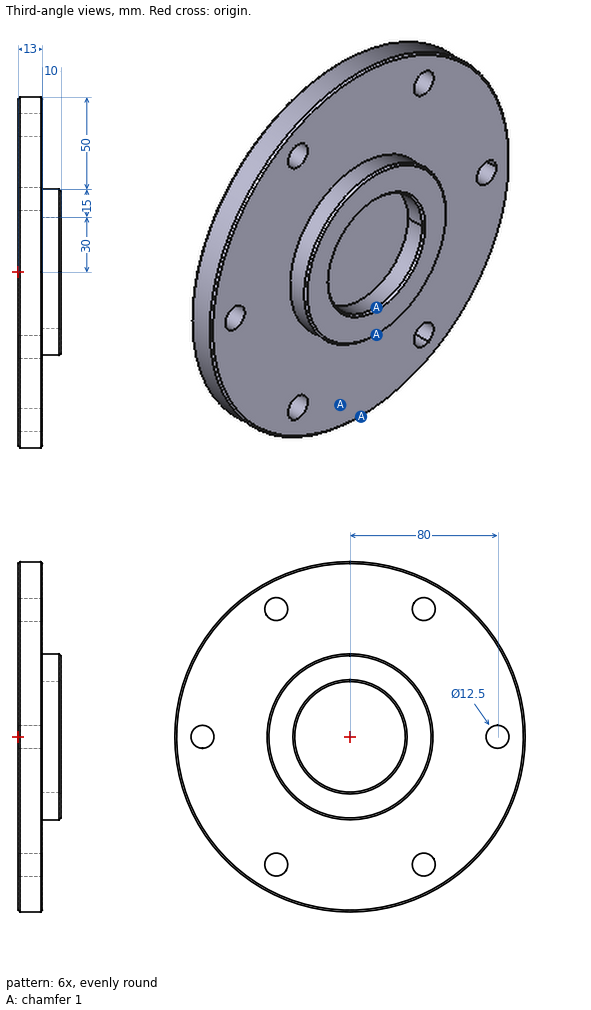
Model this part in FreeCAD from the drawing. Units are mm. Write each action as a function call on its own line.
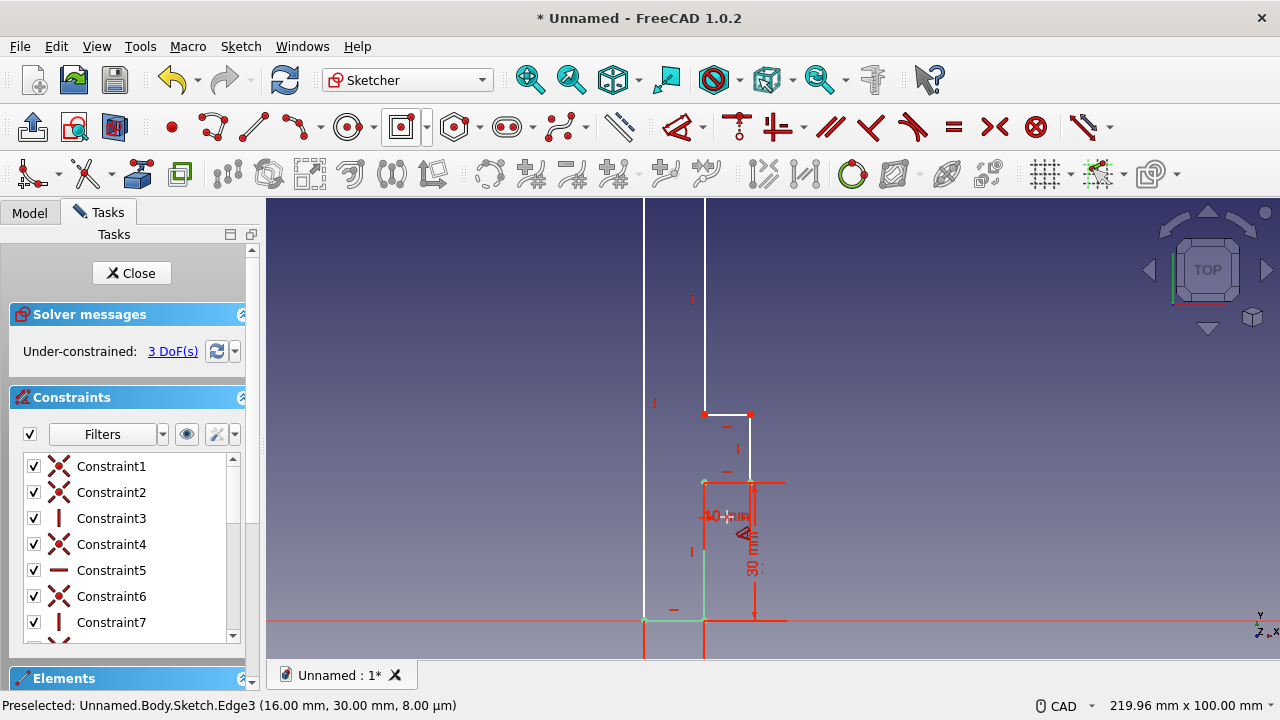
click(750, 462)
click(784, 449)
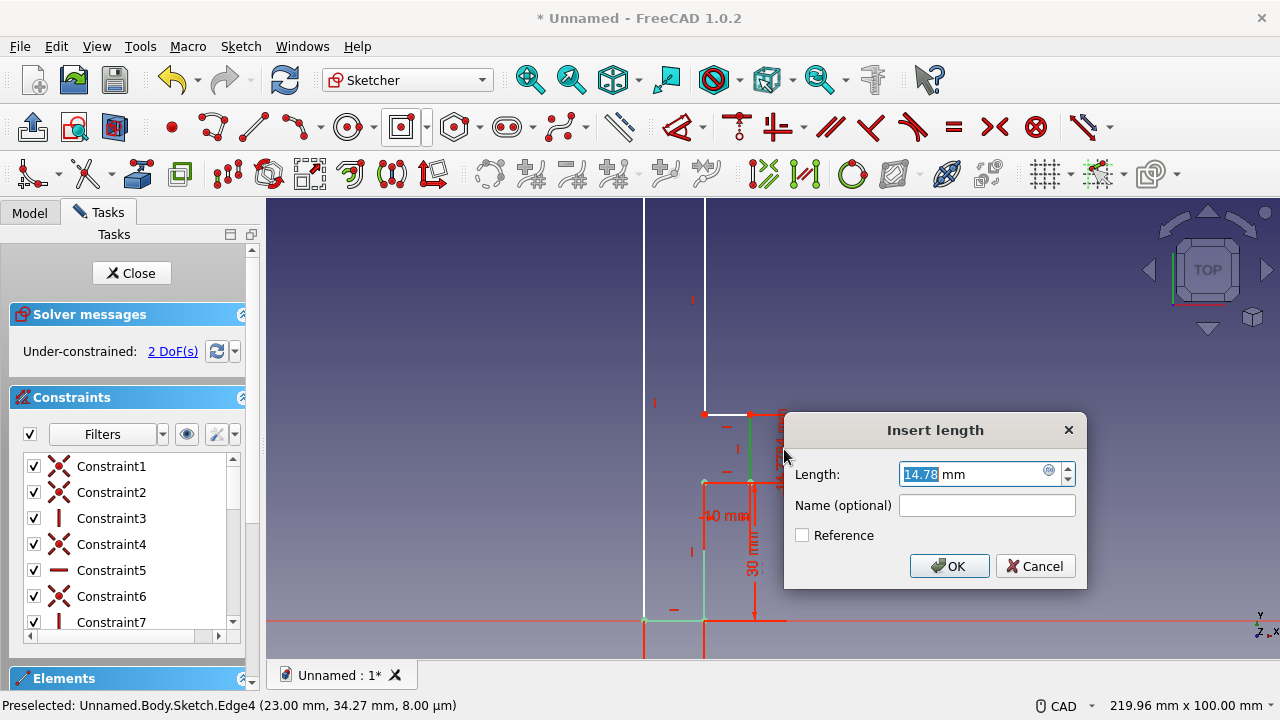
text(15)
key(Return)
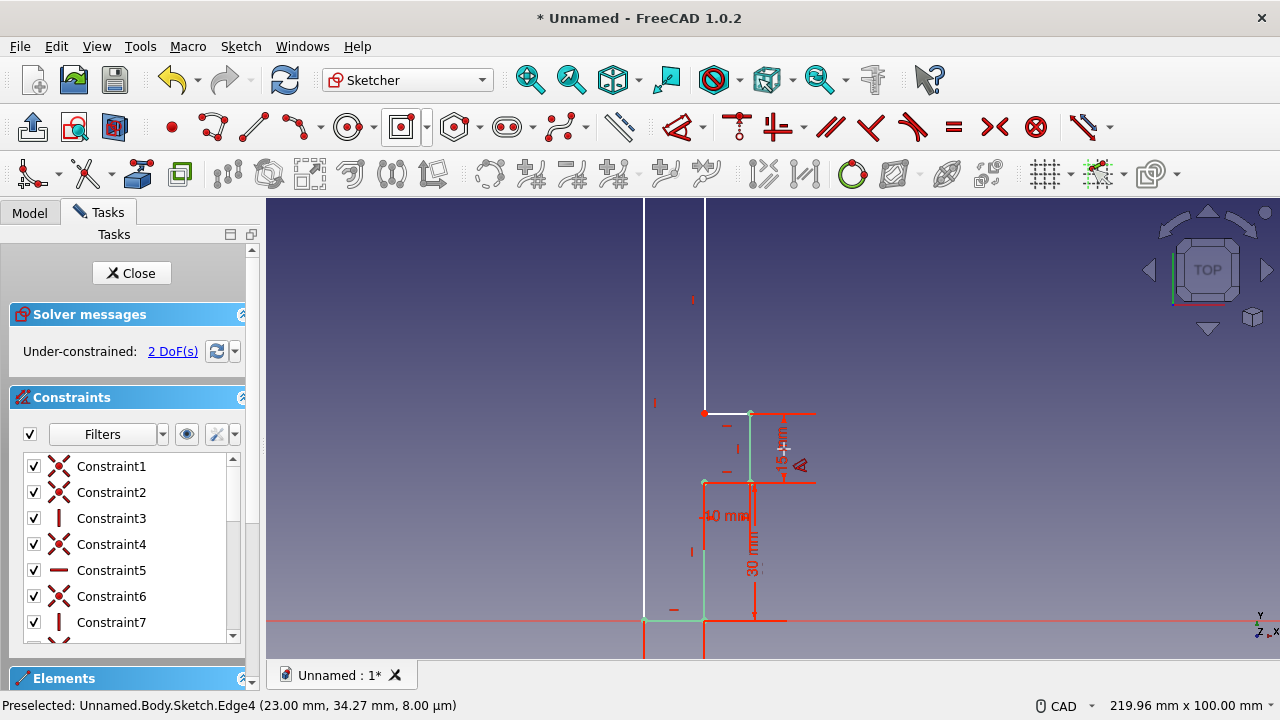
click(737, 414)
click(712, 448)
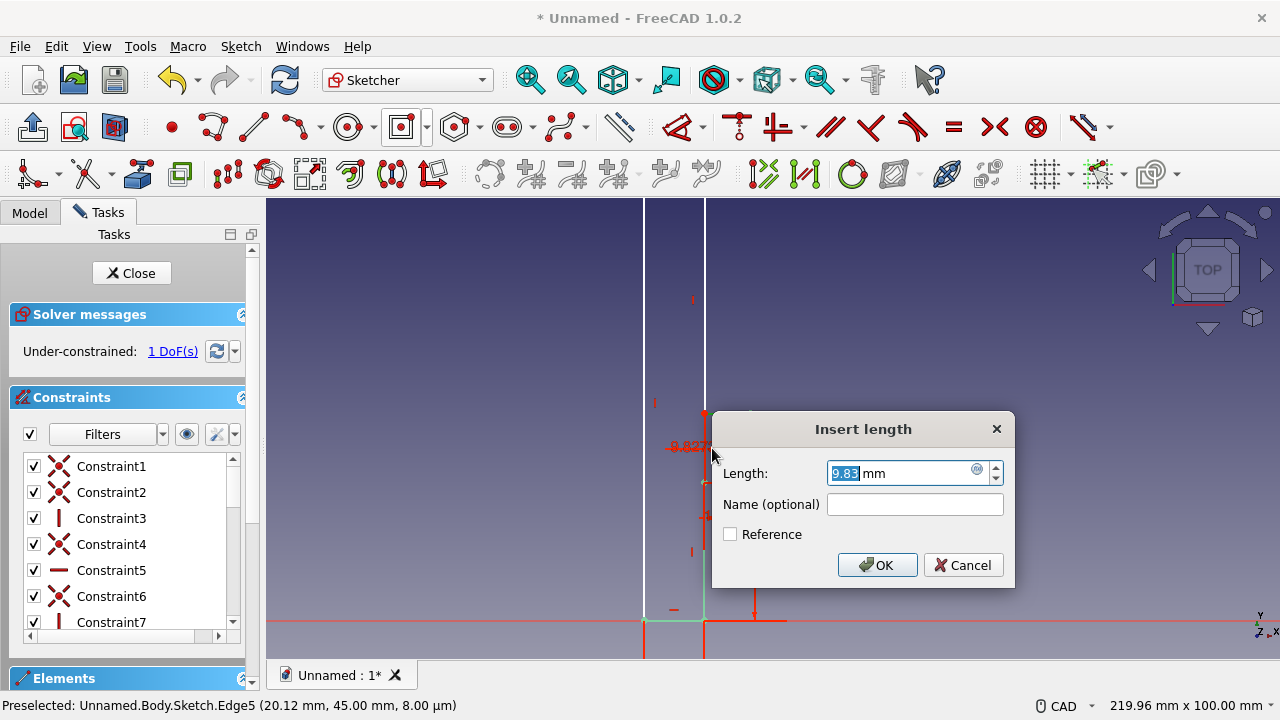
text(10)
key(Return)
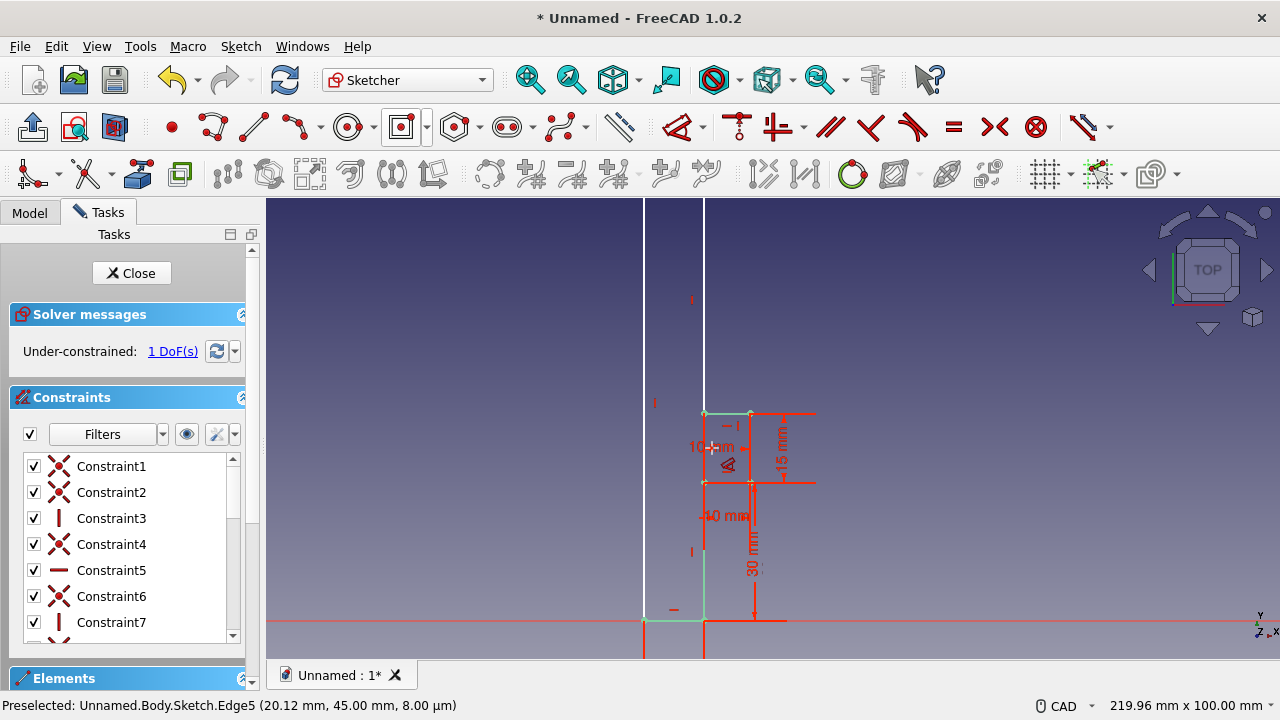
click(704, 345)
click(738, 320)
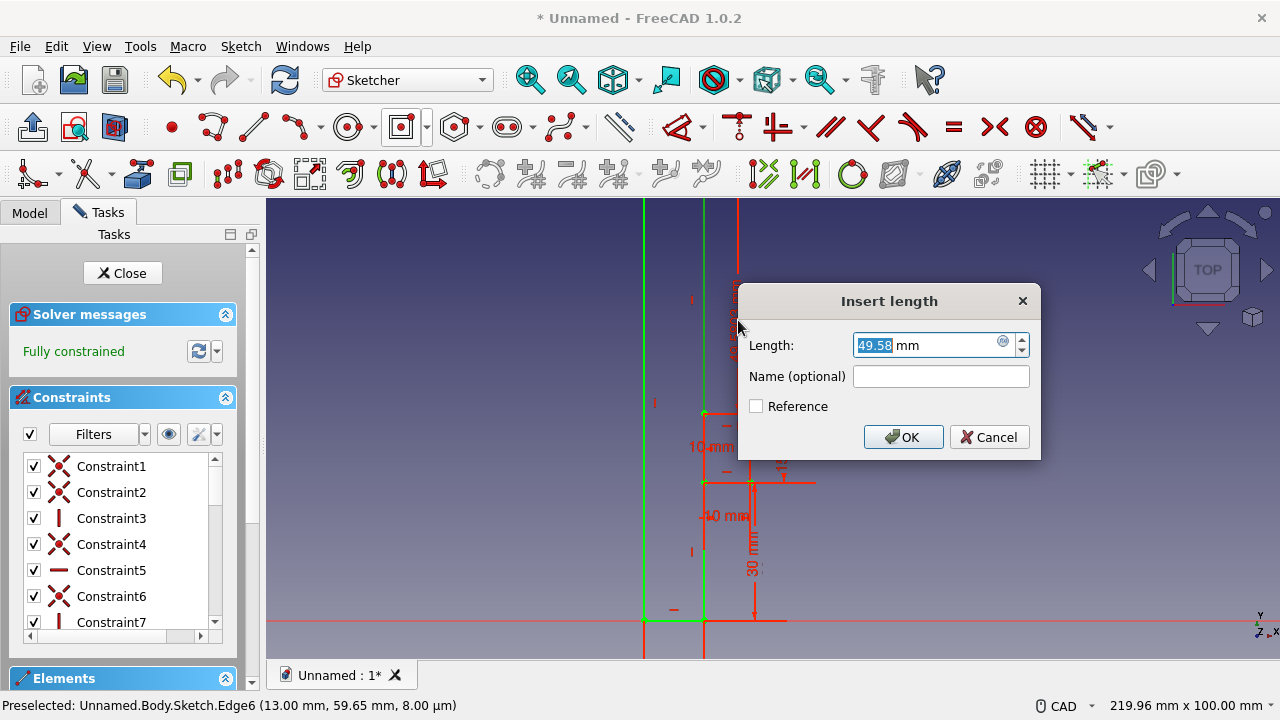
text(50)
key(Return)
key(Escape)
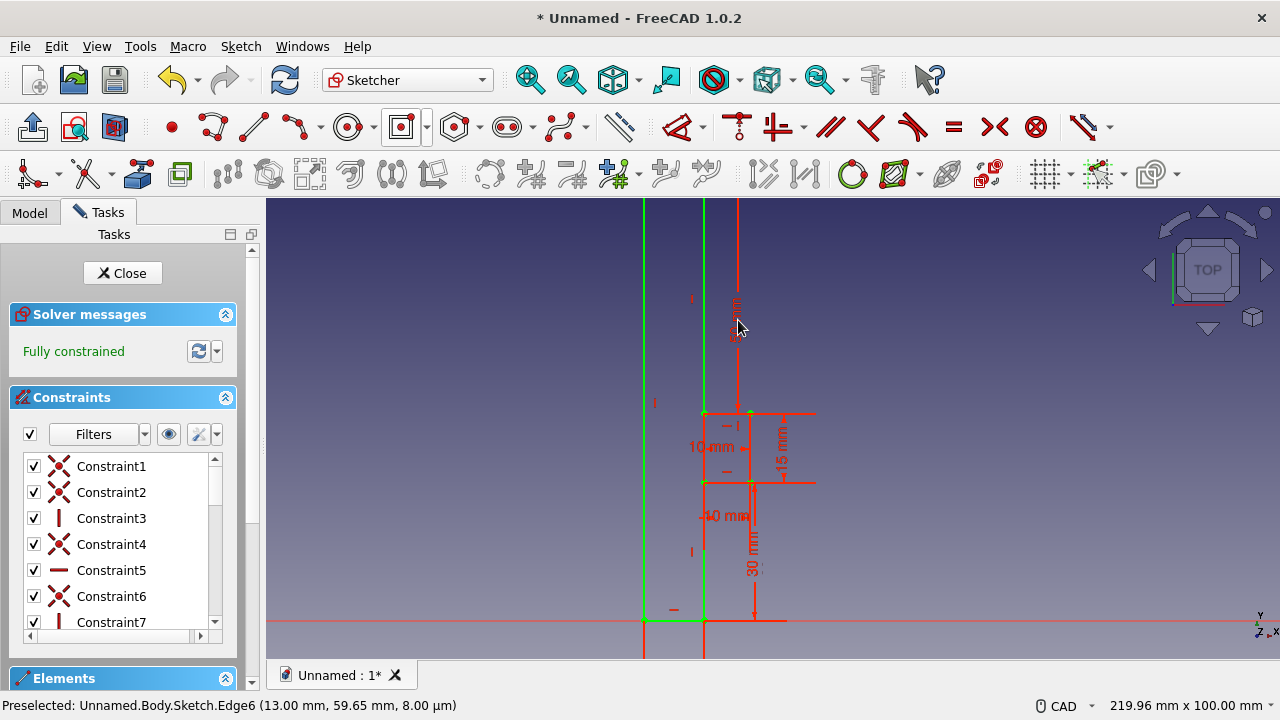
click(123, 273)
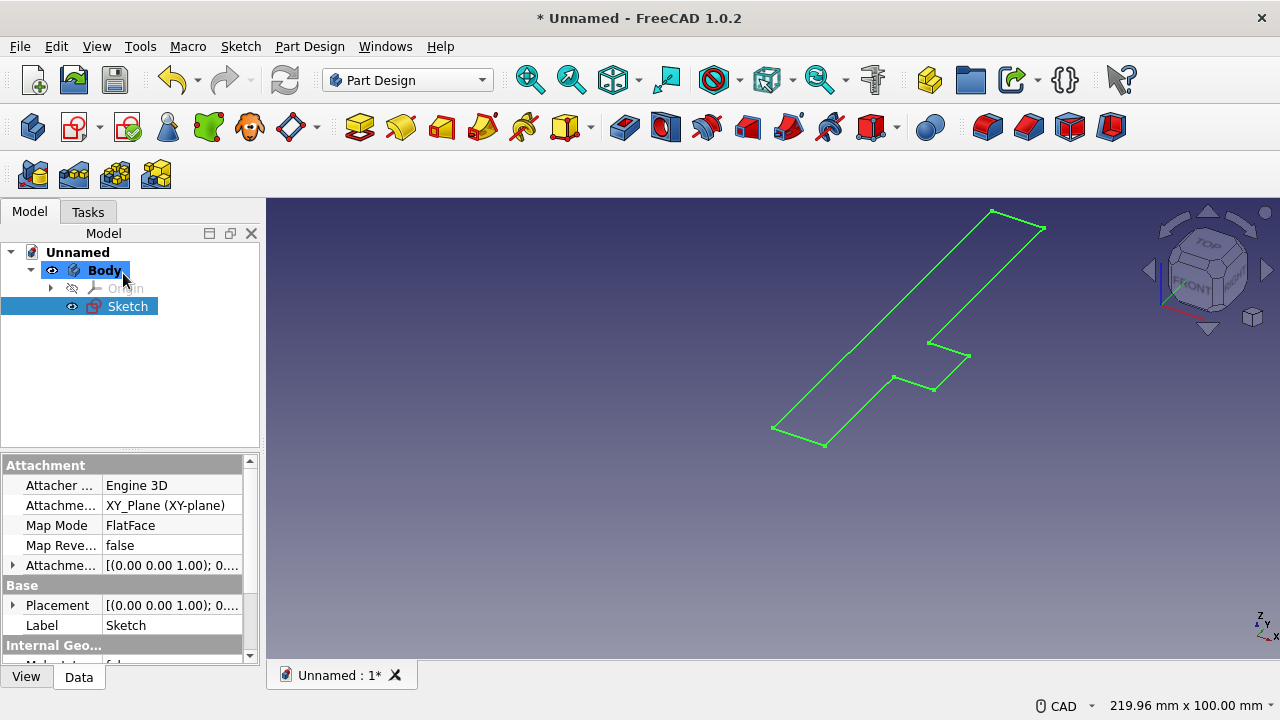
click(401, 128)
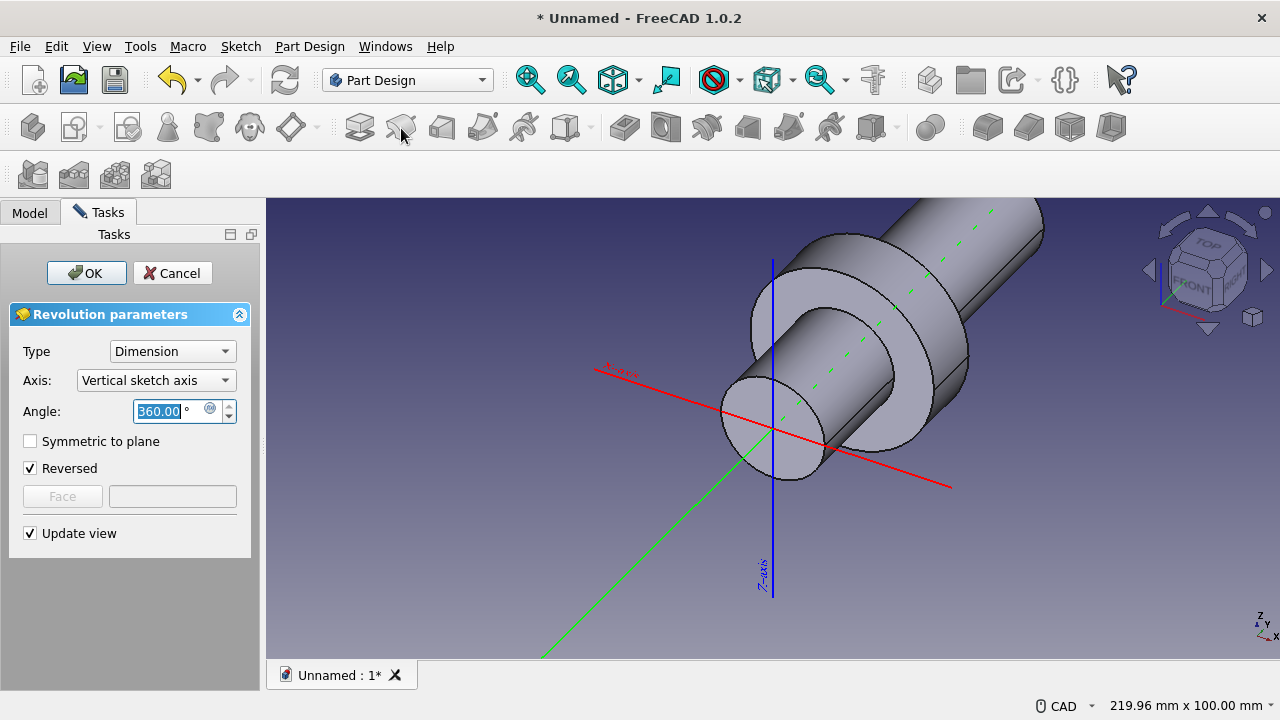
click(157, 380)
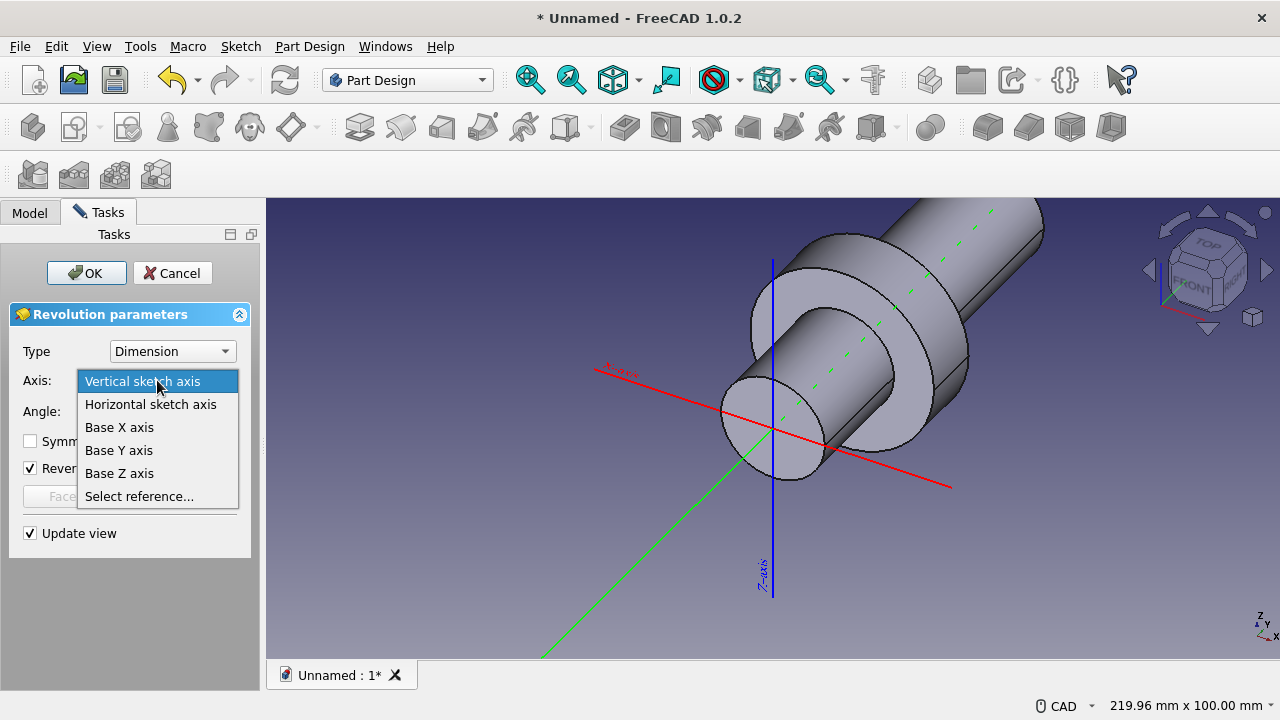
click(156, 404)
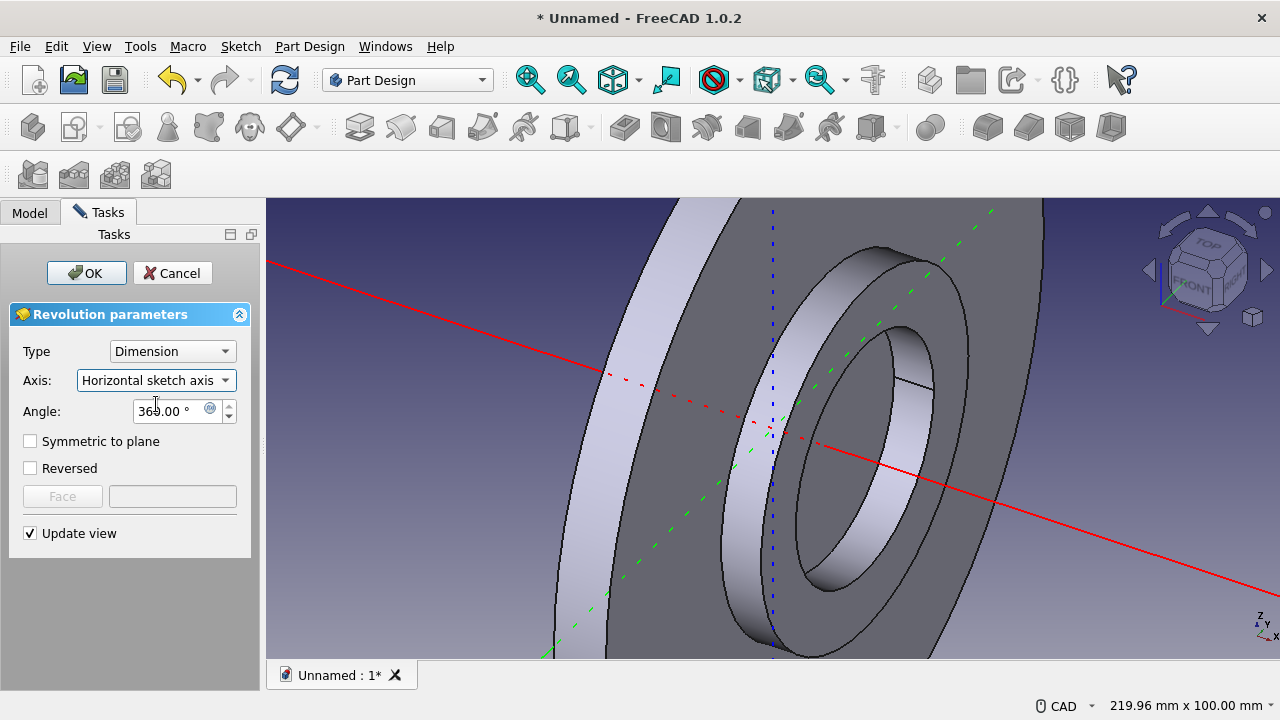
click(87, 273)